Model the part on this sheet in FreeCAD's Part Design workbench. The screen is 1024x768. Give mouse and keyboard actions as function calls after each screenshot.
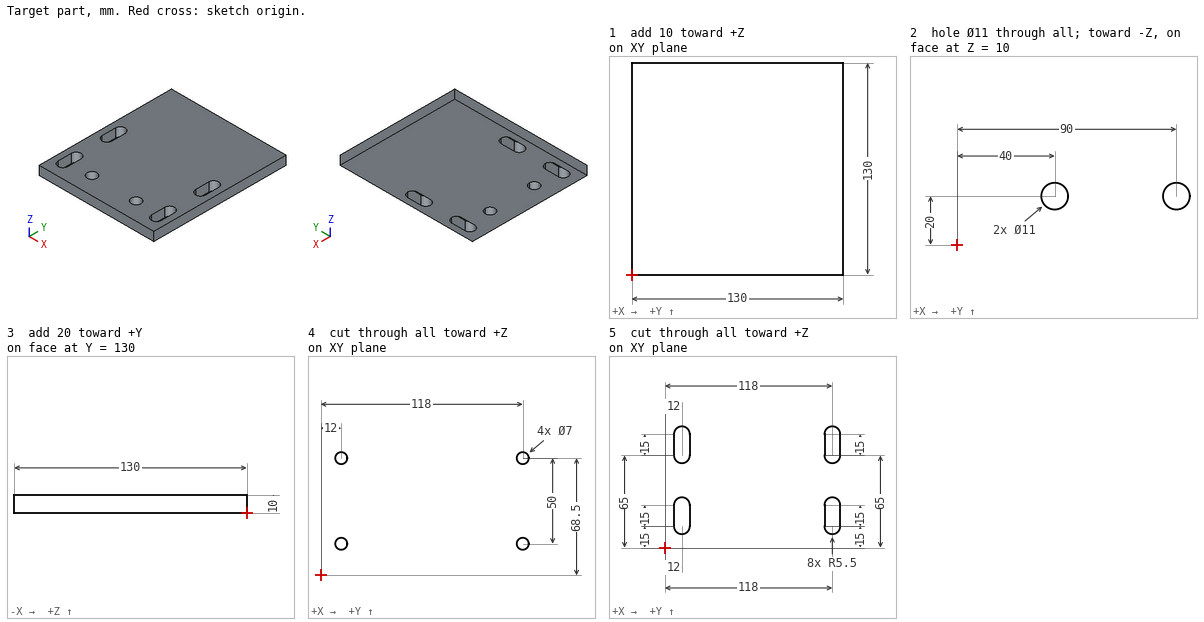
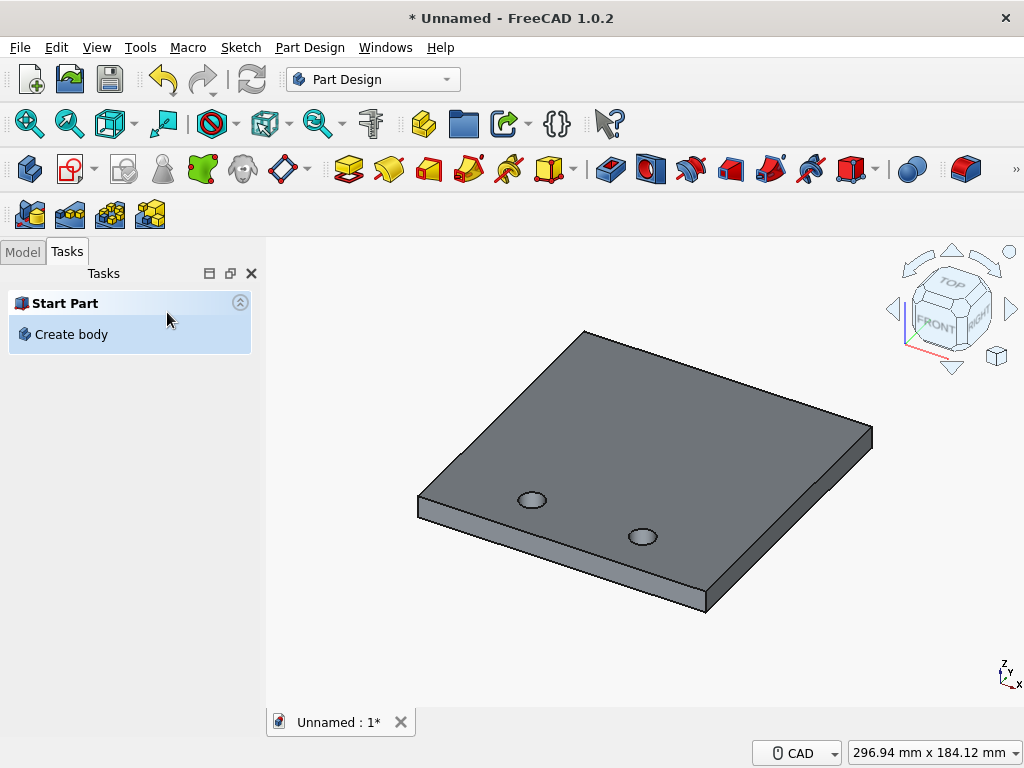
key(4)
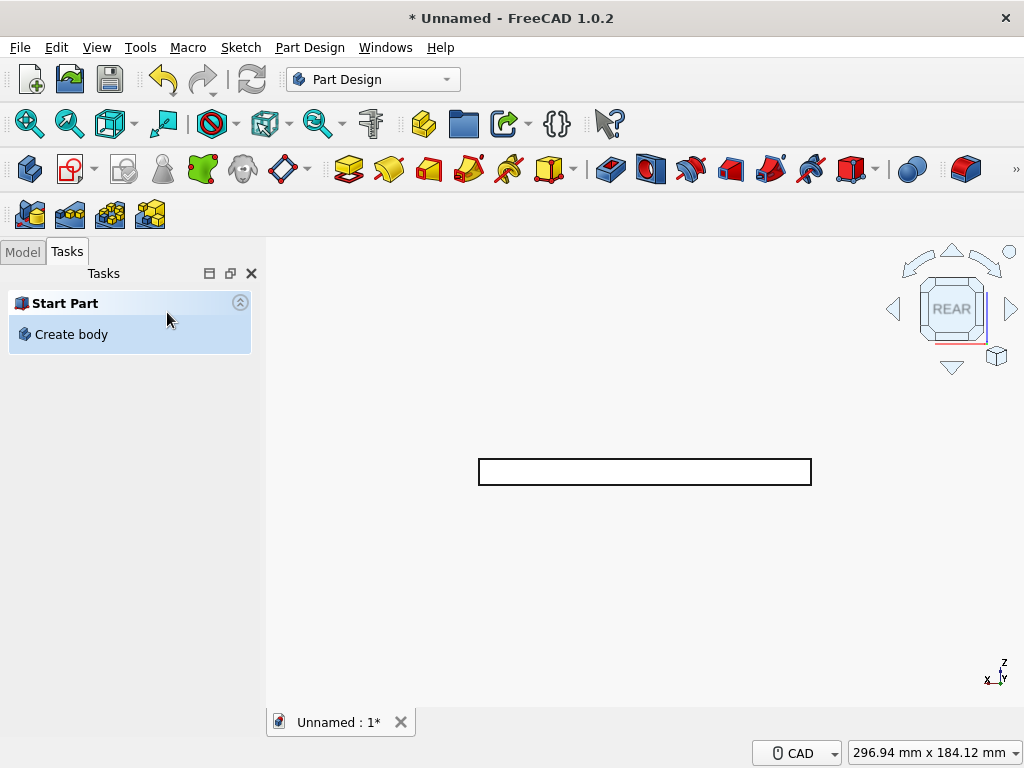
click(30, 124)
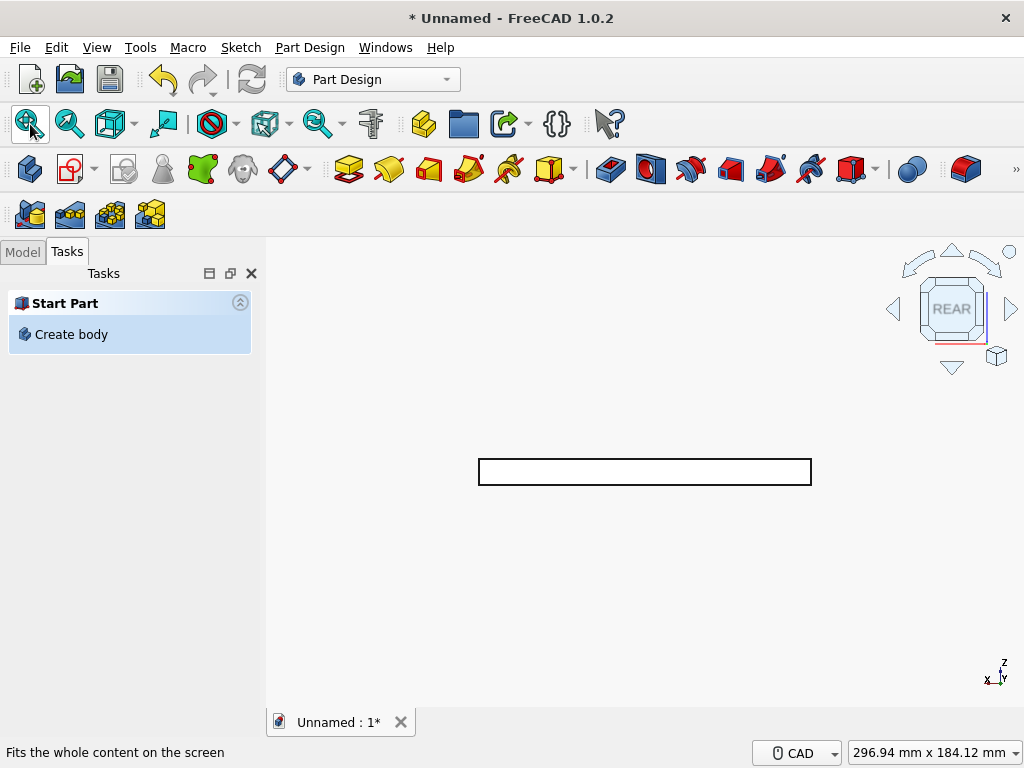
click(503, 471)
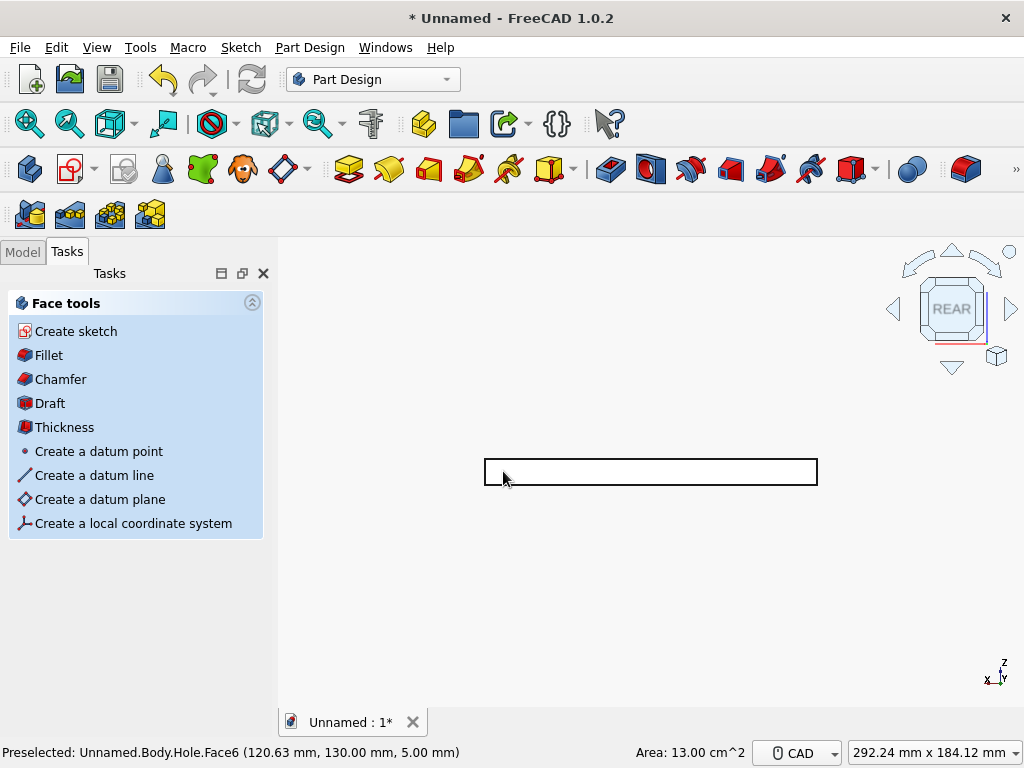
click(70, 170)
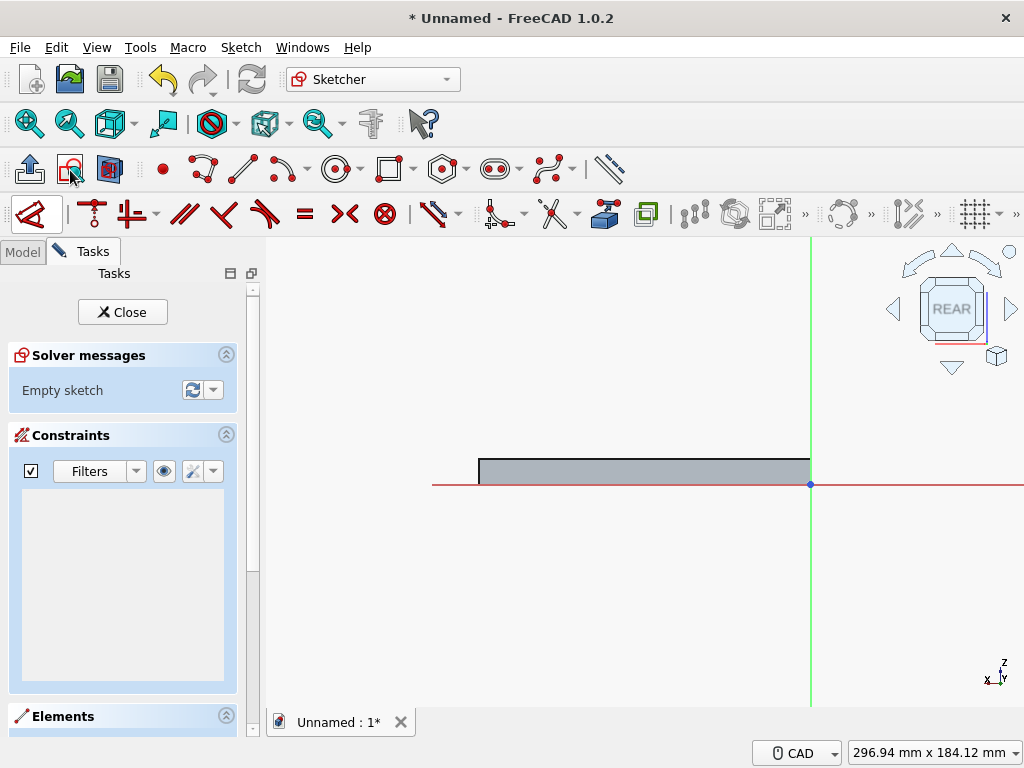
click(390, 170)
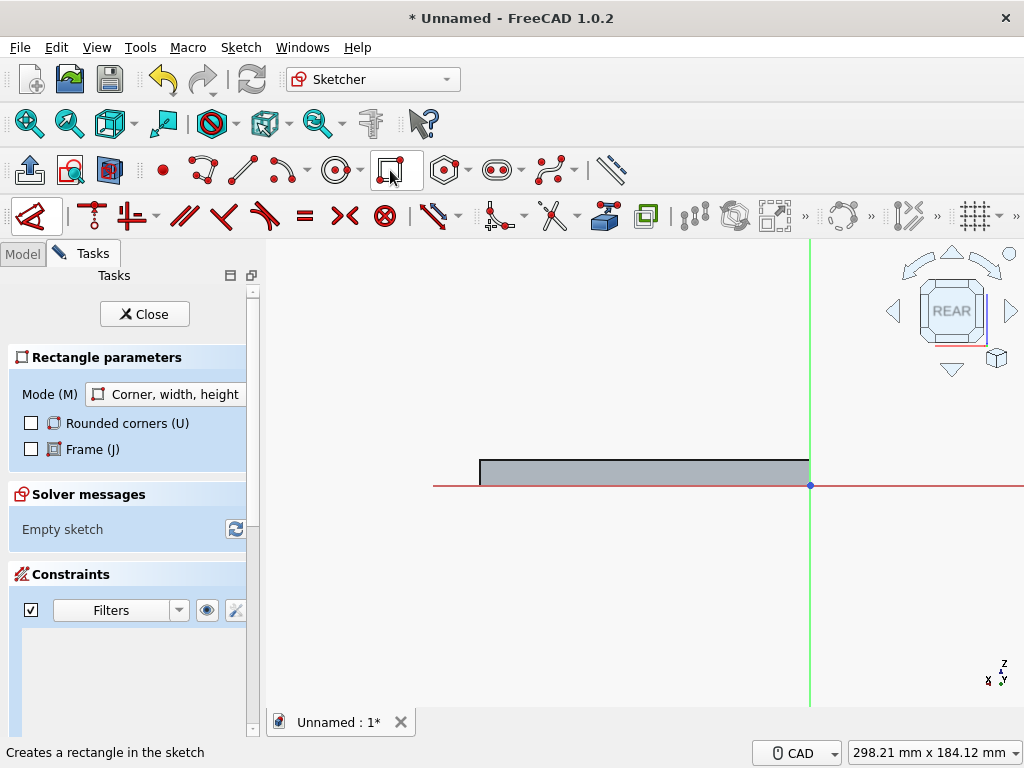
click(810, 486)
click(480, 460)
key(Escape)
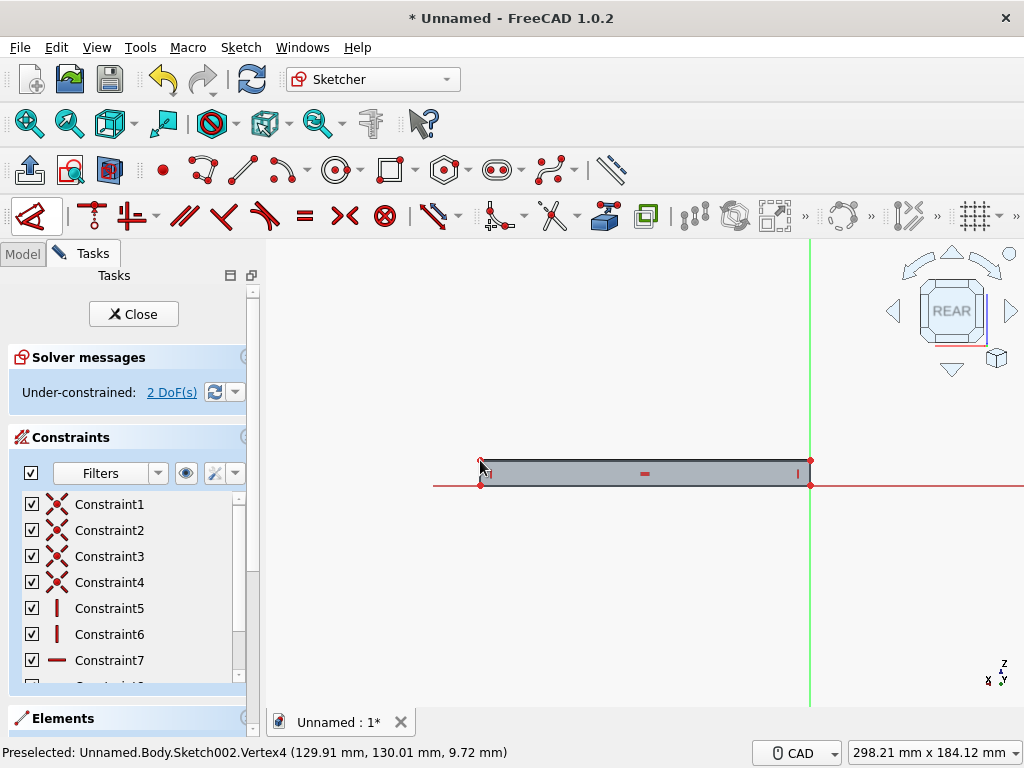
scroll(810, 476, up, 3)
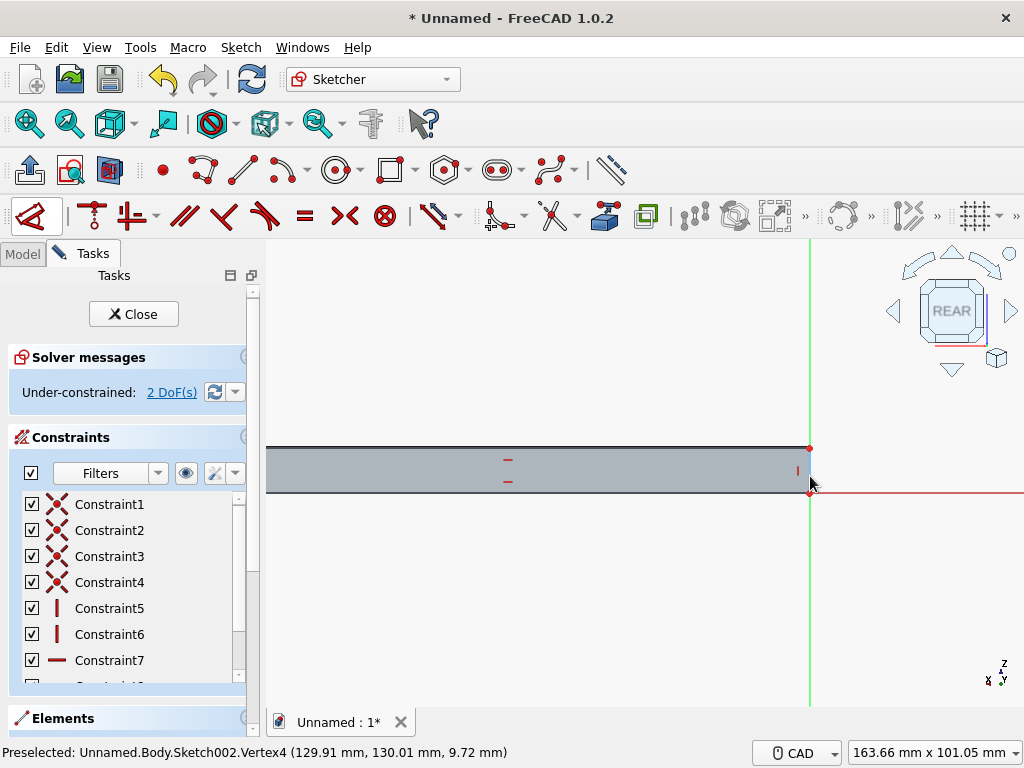
click(810, 475)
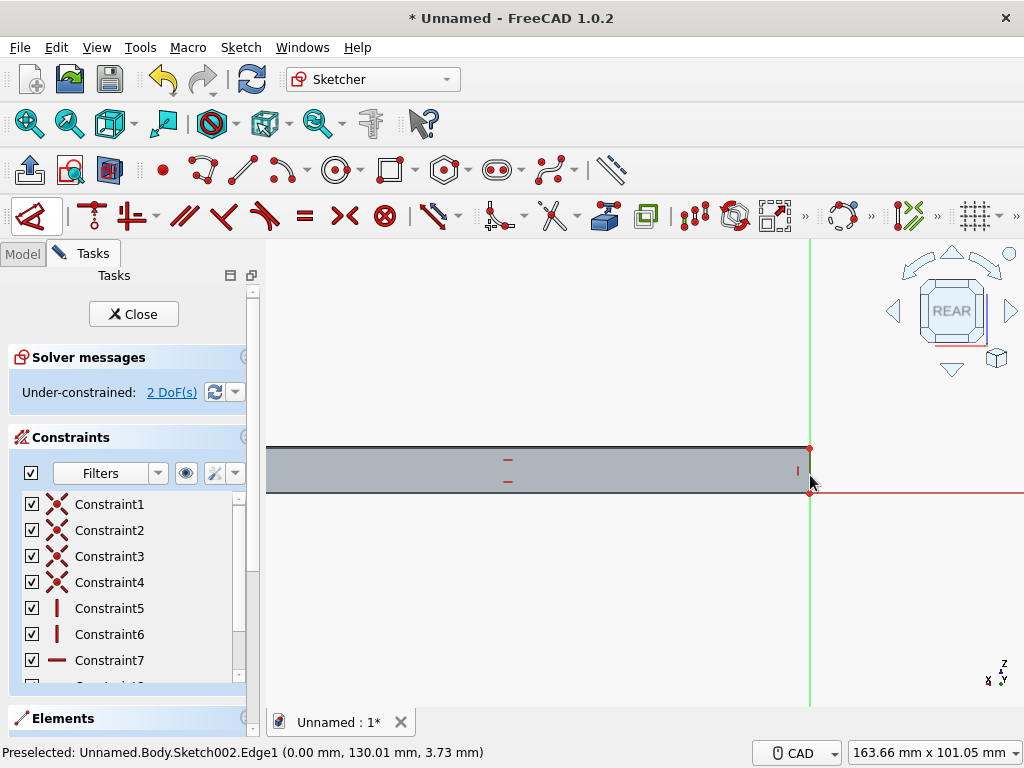
key(i)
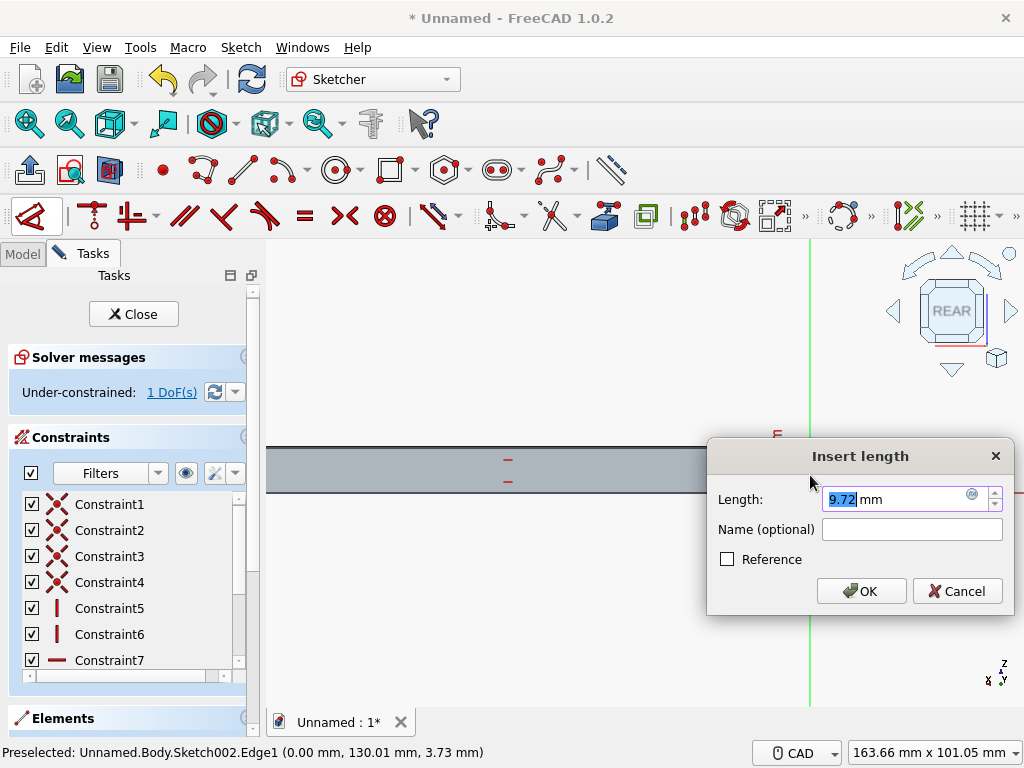
text(10)
key(Return)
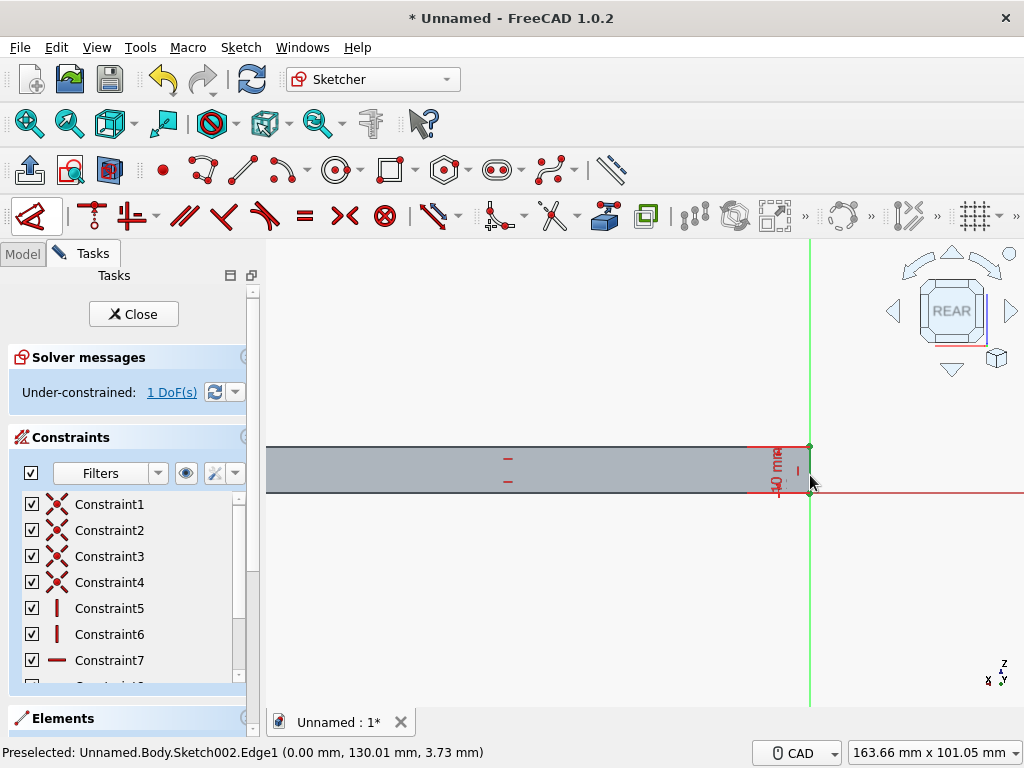
click(629, 447)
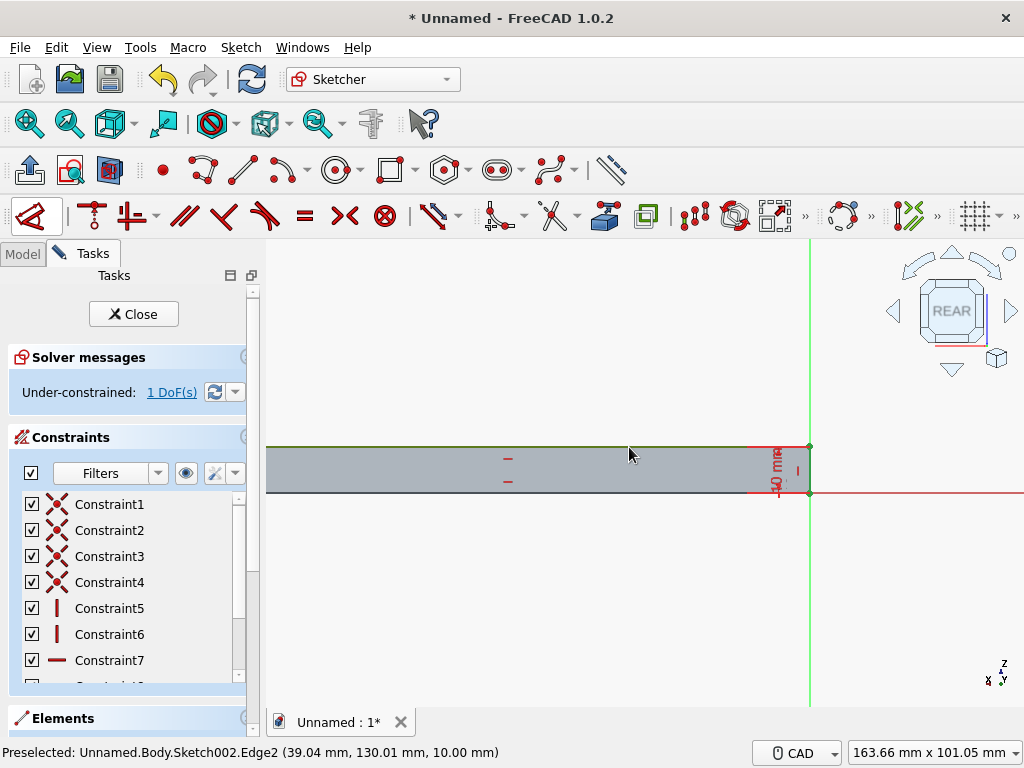
click(56, 216)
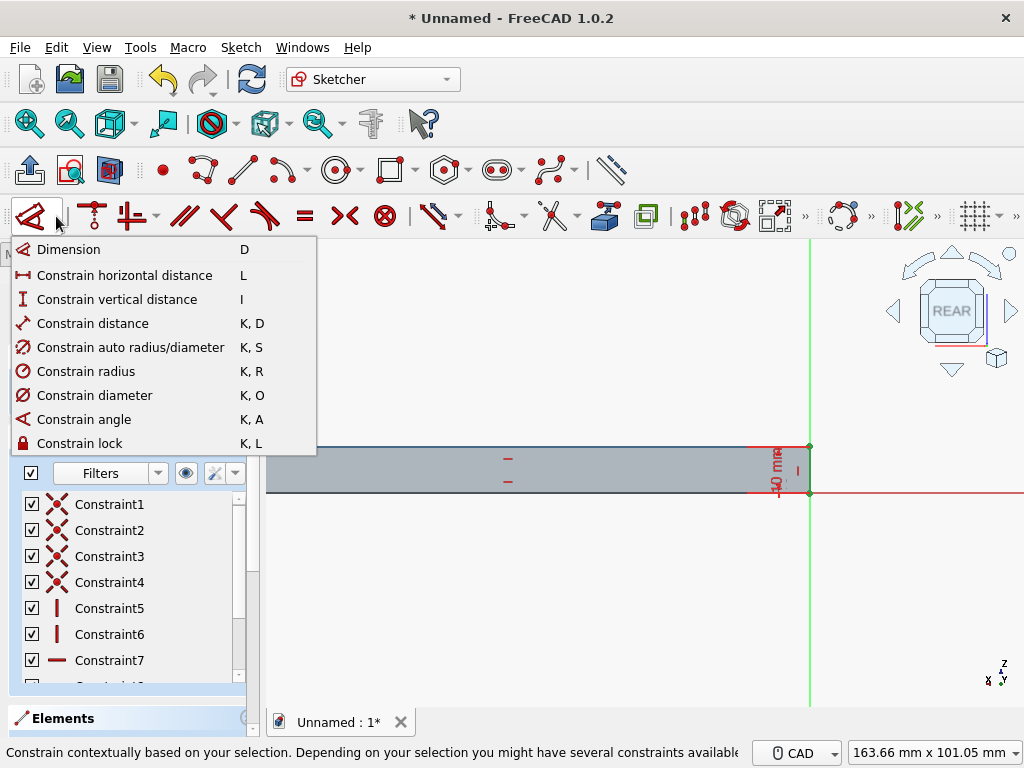
click(164, 275)